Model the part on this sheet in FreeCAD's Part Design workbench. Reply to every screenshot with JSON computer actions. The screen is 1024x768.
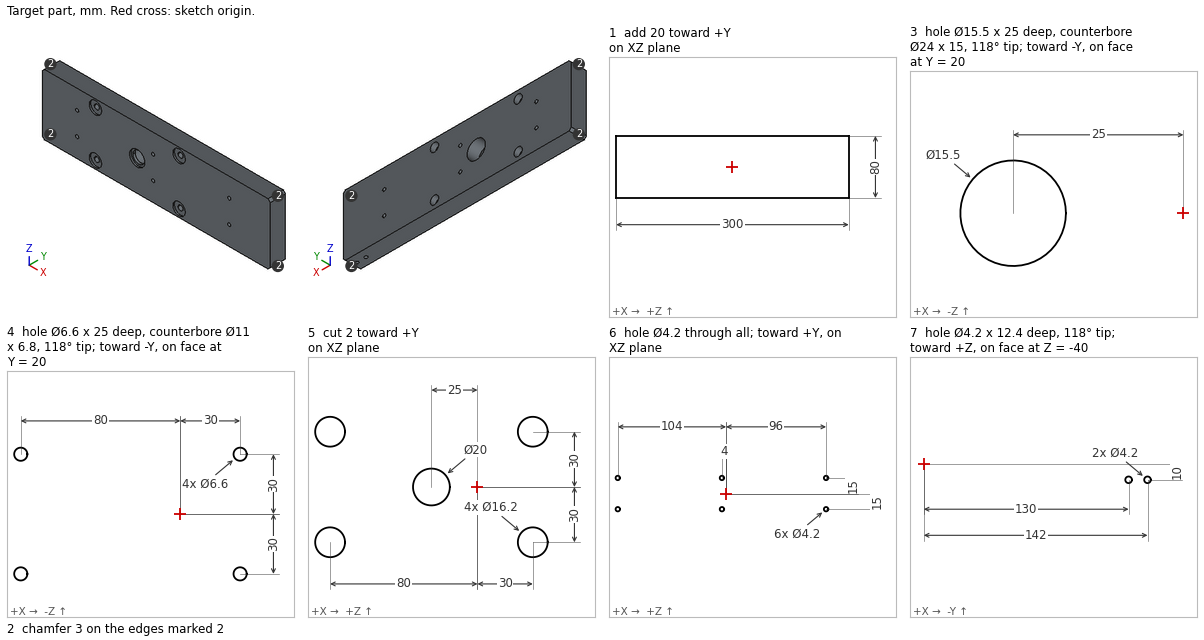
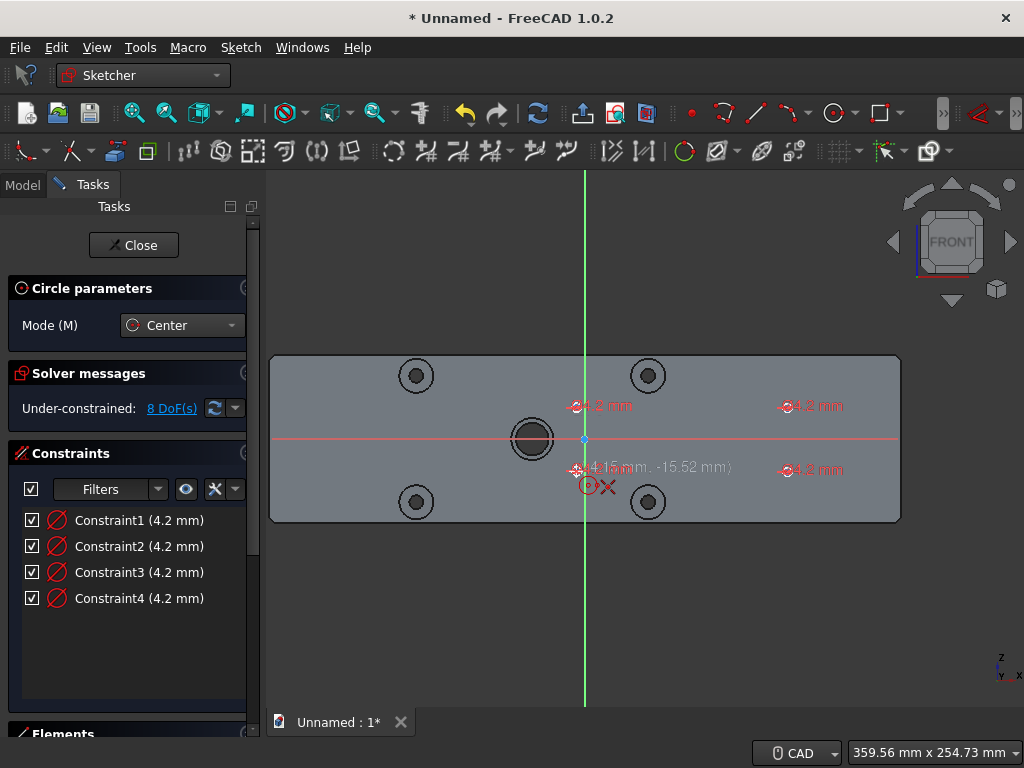
{"action": "scroll", "coordinate": [366, 407], "scroll_direction": "up", "scroll_amount": 9}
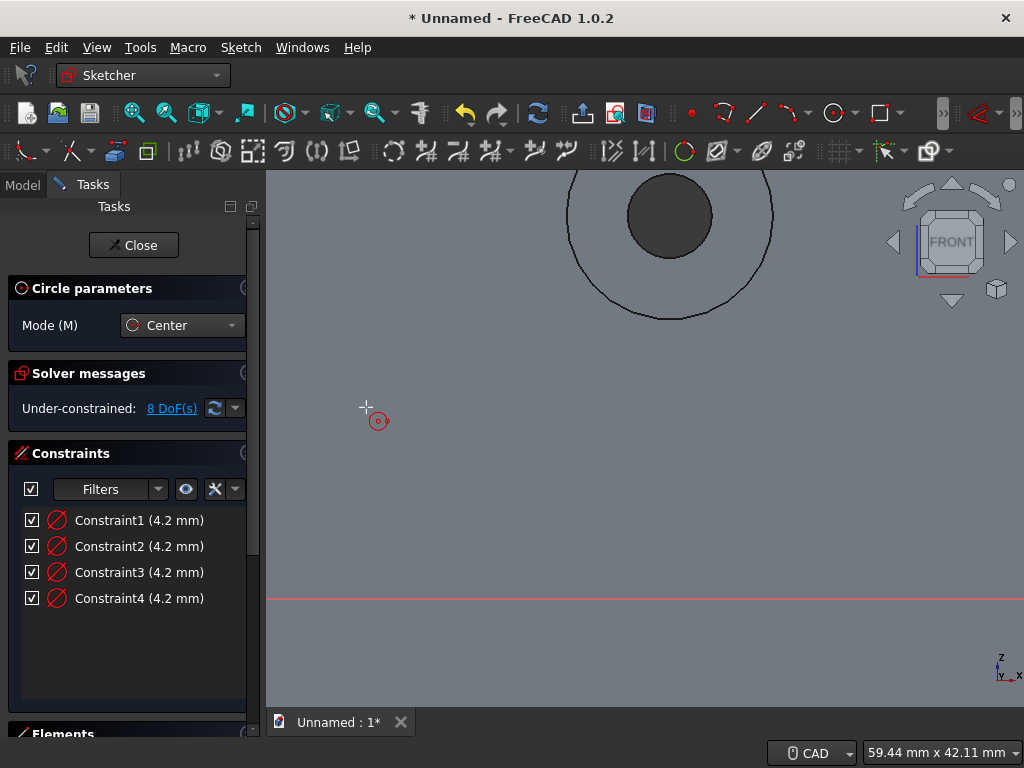
{"action": "scroll", "coordinate": [366, 407], "scroll_direction": "down", "scroll_amount": 9}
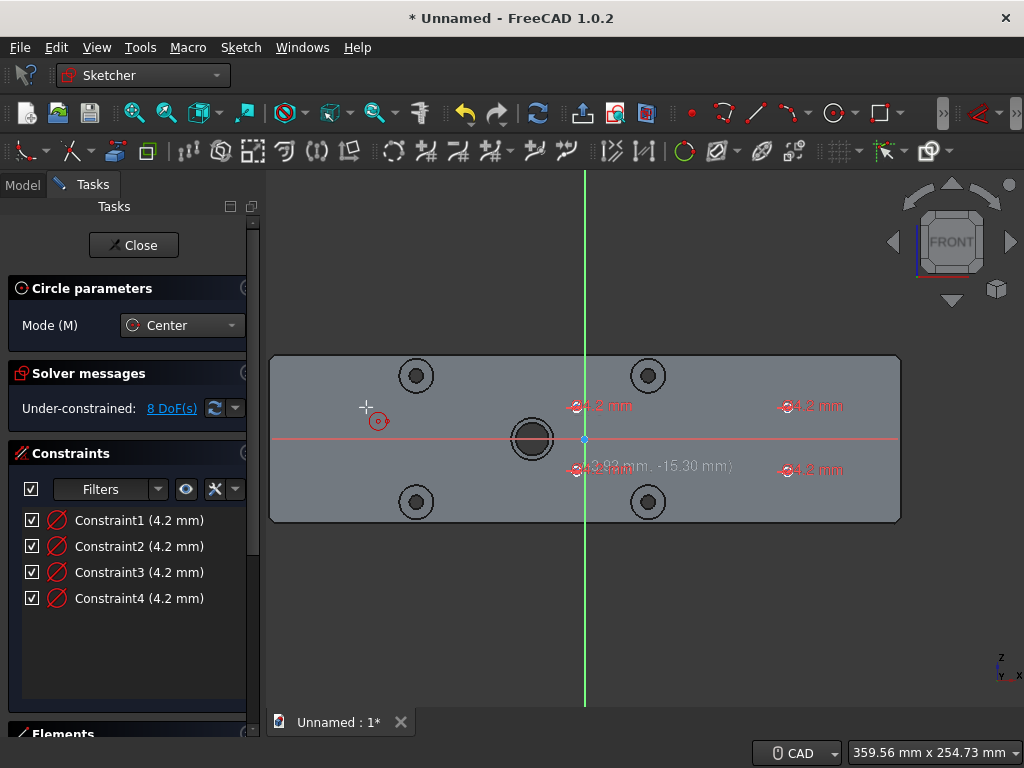
{"action": "left_click", "coordinate": [366, 407]}
{"action": "mouse_move", "coordinate": [369, 404]}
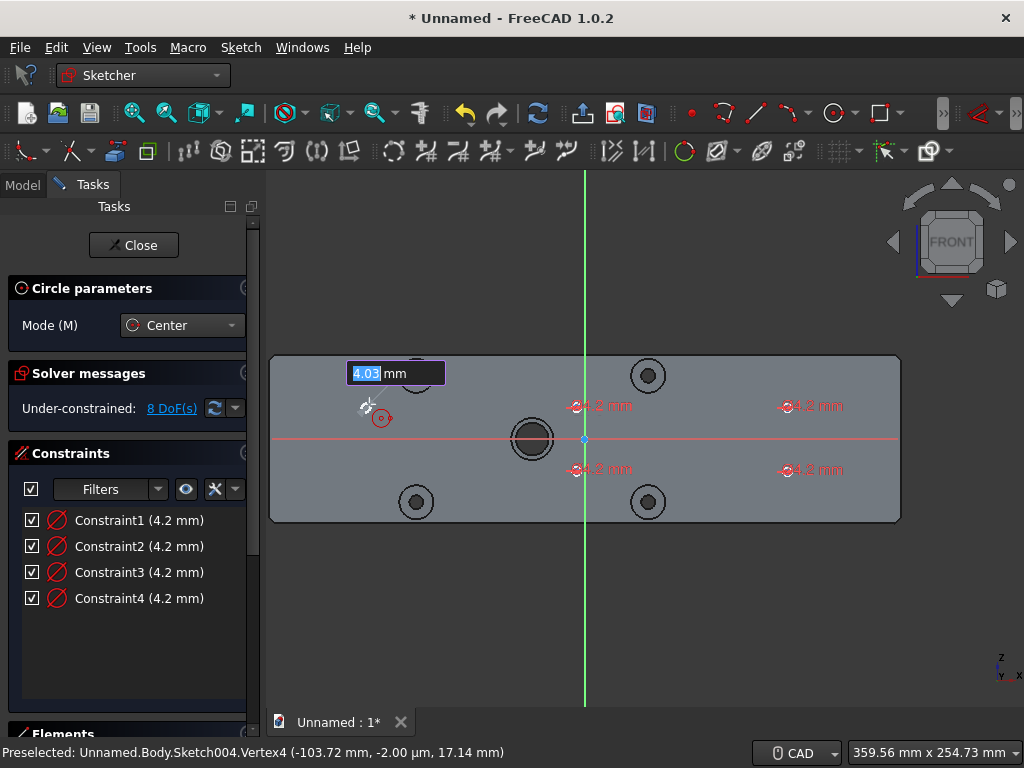
{"action": "type", "text": "4.2"}
{"action": "key", "text": "Return"}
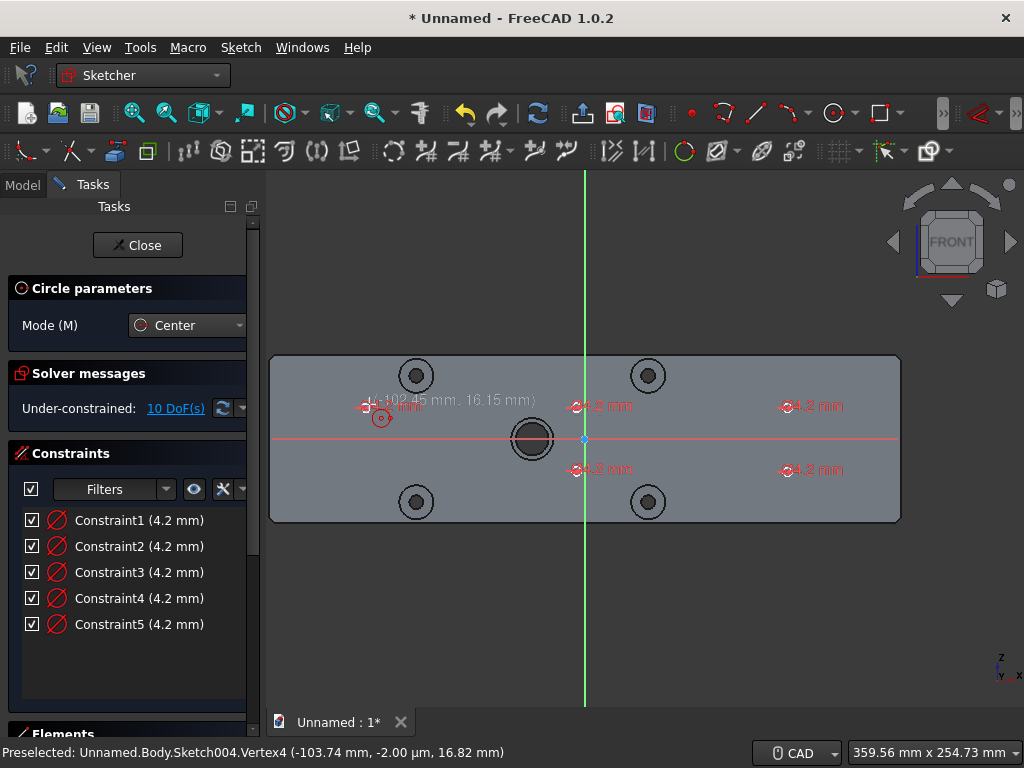
{"action": "scroll", "coordinate": [366, 471], "scroll_direction": "up", "scroll_amount": 9}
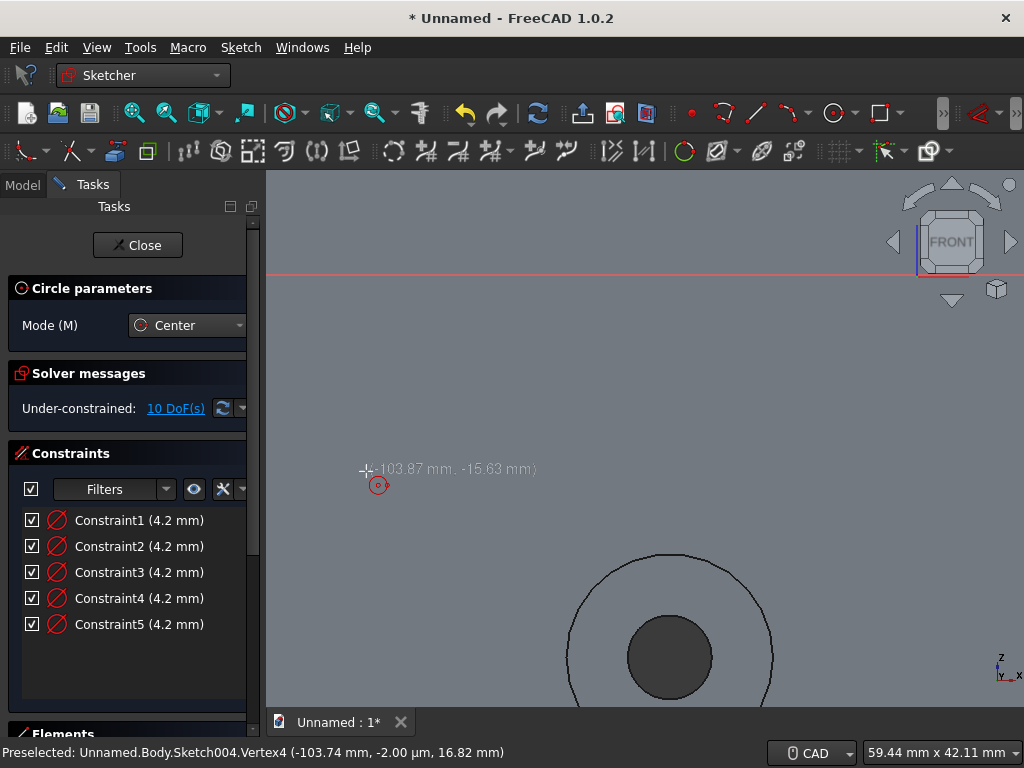
{"action": "scroll", "coordinate": [366, 471], "scroll_direction": "down", "scroll_amount": 9}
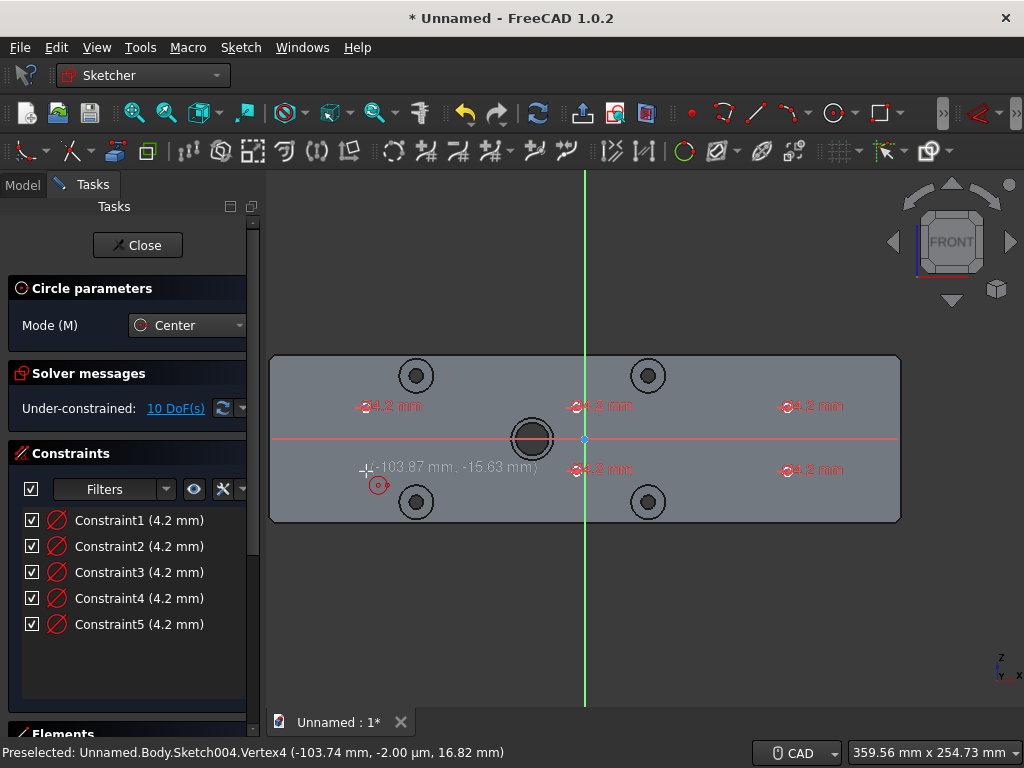
{"action": "left_click", "coordinate": [366, 471]}
{"action": "mouse_move", "coordinate": [369, 468]}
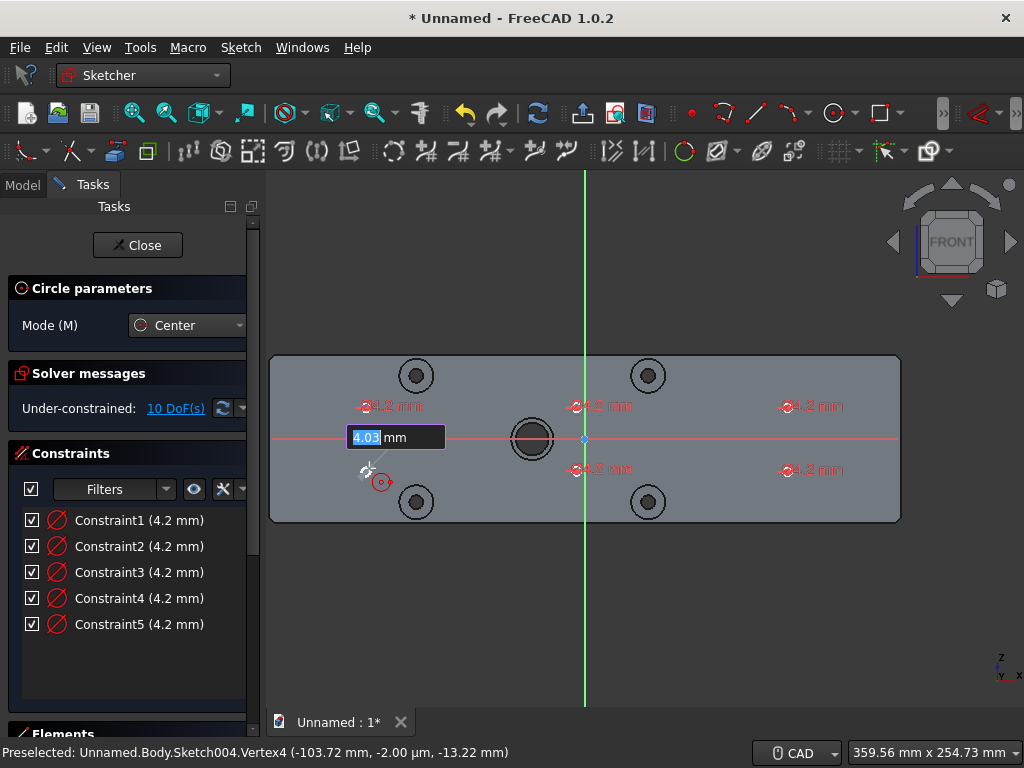
{"action": "type", "text": "4.2"}
{"action": "key", "text": "Return"}
{"action": "key", "text": "Escape"}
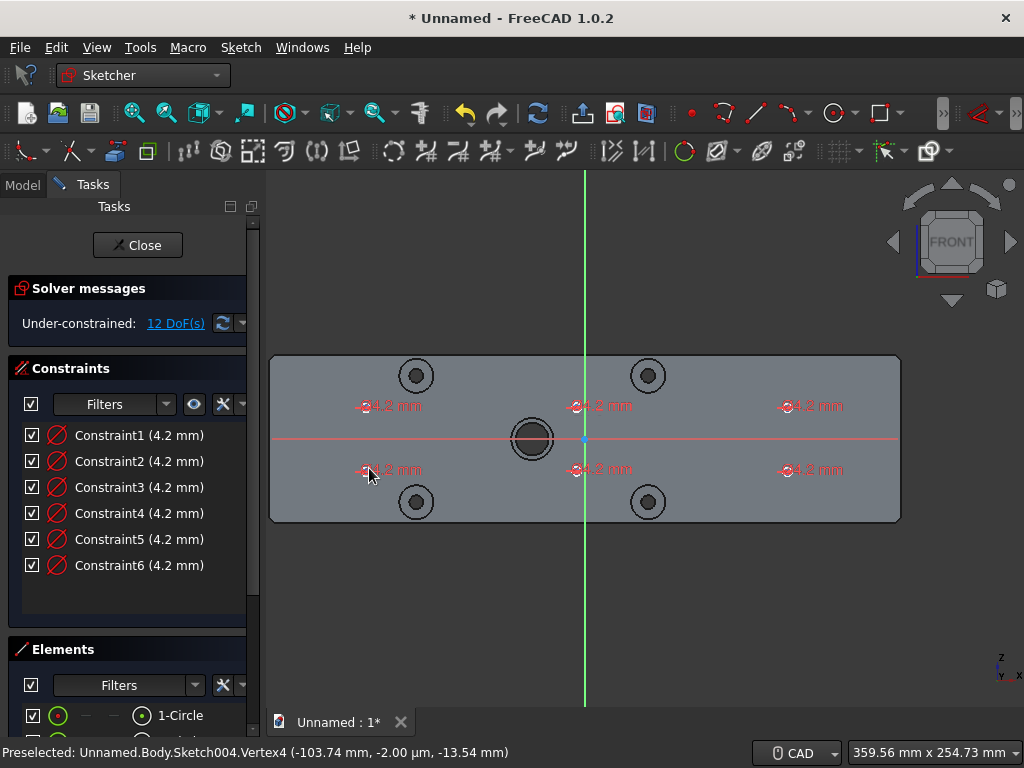
{"action": "left_click", "coordinate": [787, 408]}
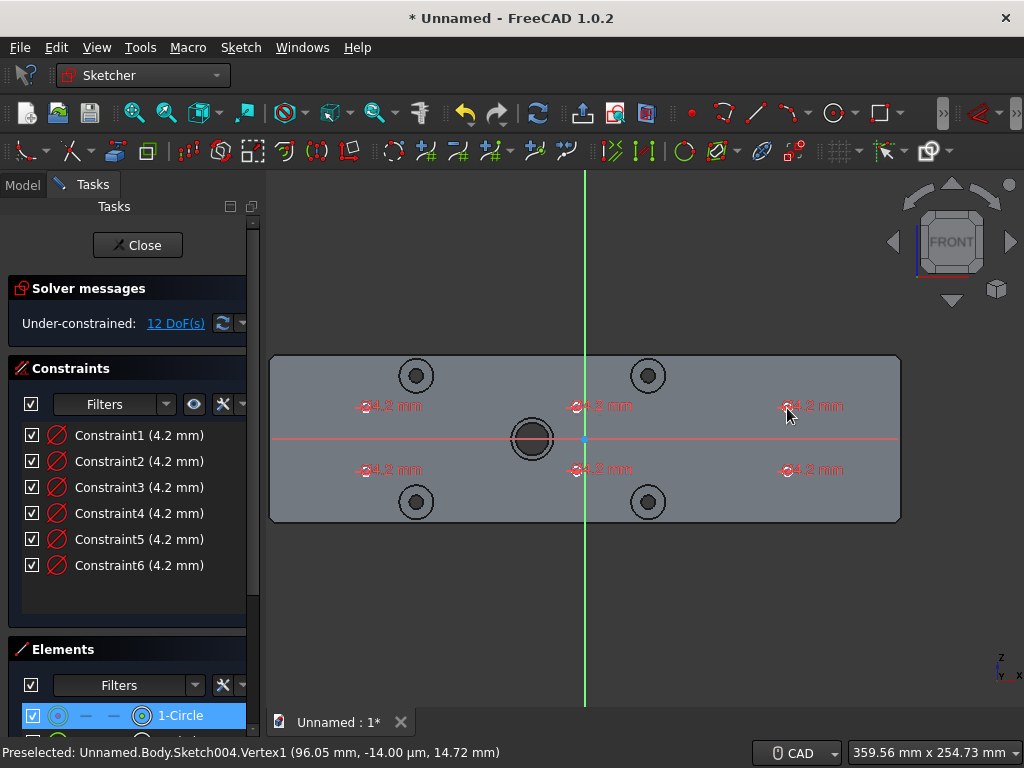
{"action": "left_click", "coordinate": [787, 472]}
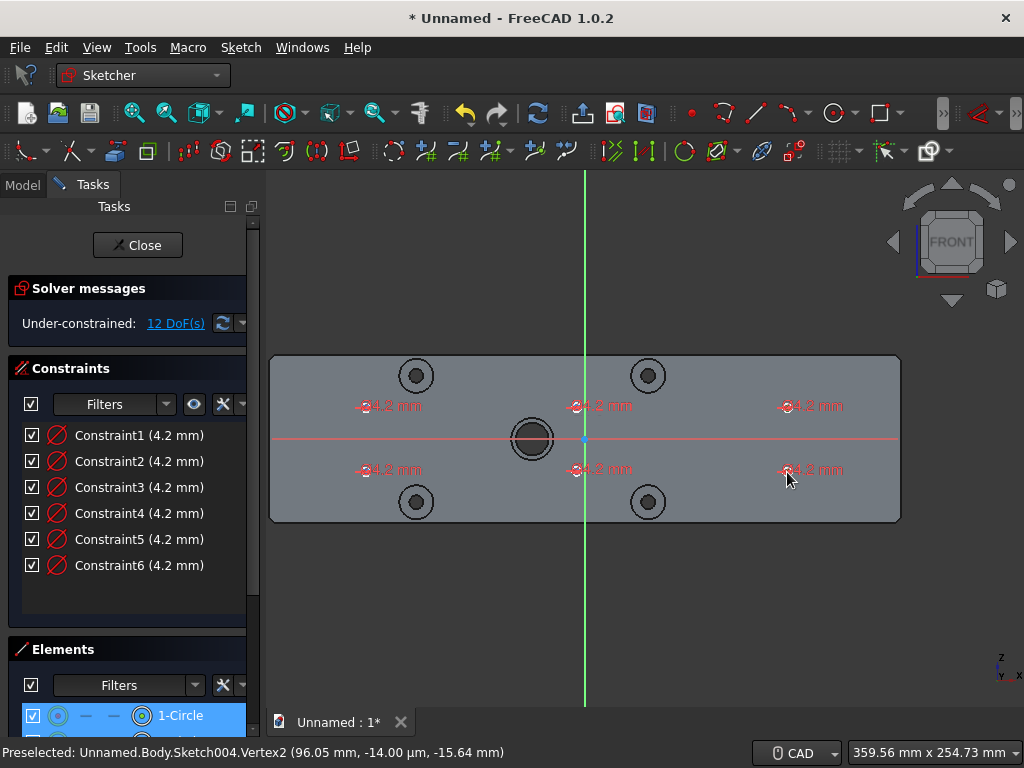
{"action": "key", "text": "v"}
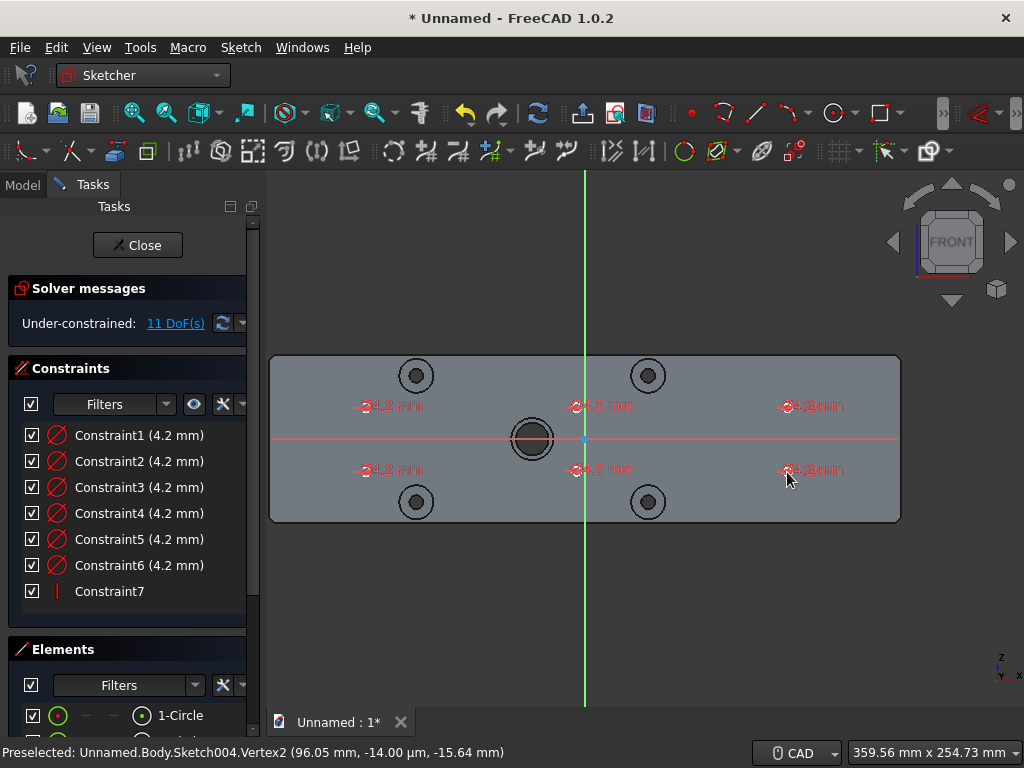
{"action": "left_click", "coordinate": [787, 408]}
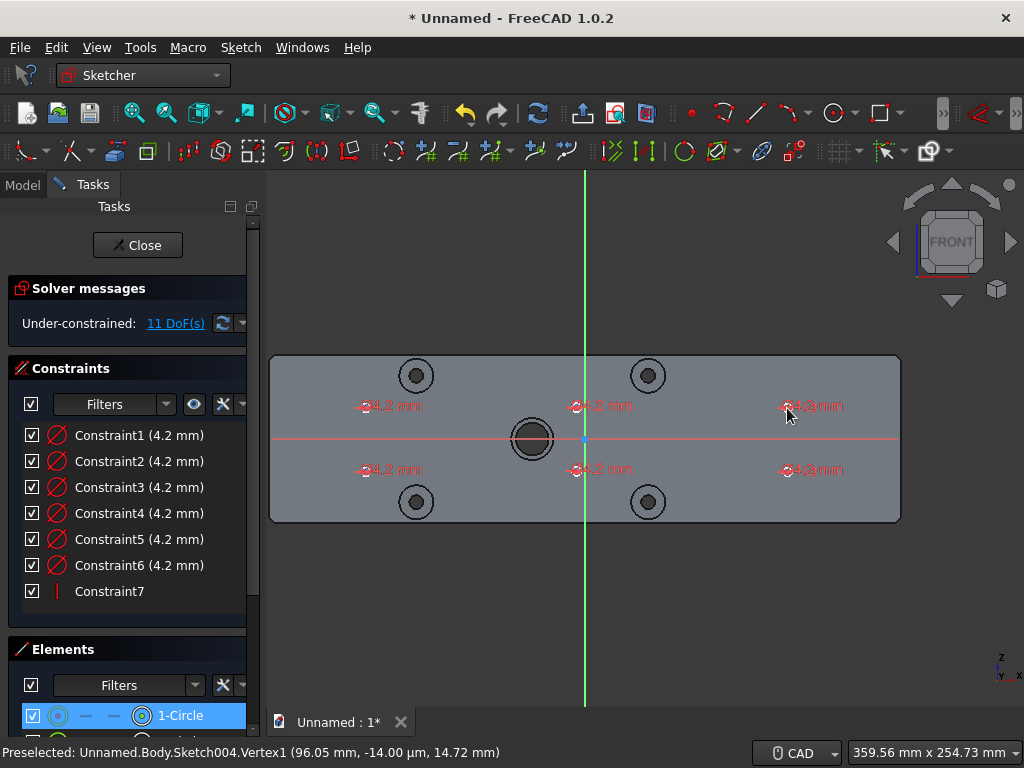
{"action": "left_click", "coordinate": [577, 408]}